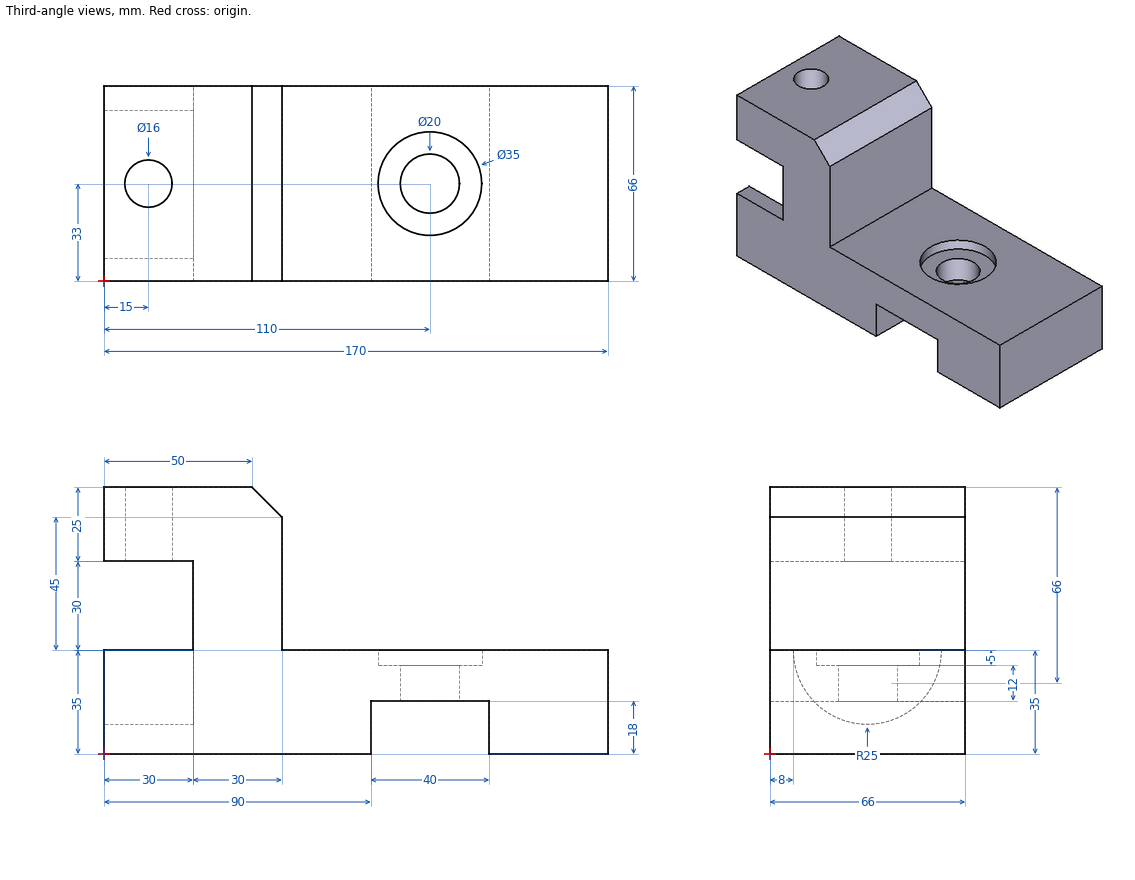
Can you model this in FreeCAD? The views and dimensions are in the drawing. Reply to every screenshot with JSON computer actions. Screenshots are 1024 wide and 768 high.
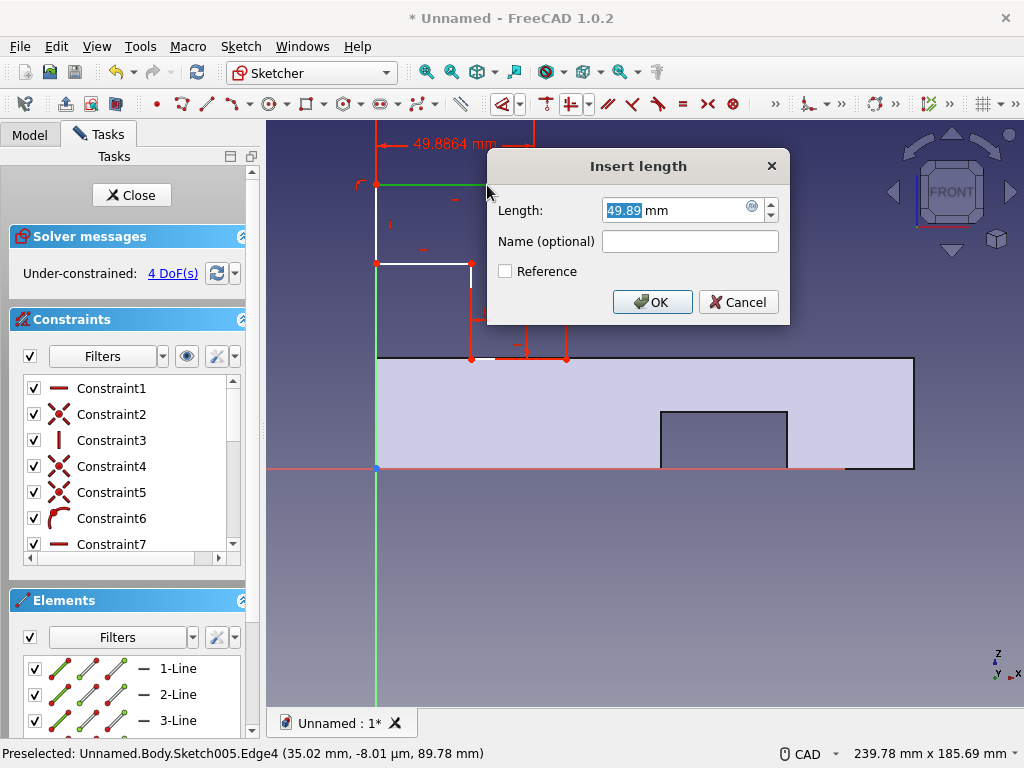
{"action": "type", "text": "50"}
{"action": "key", "text": "Return"}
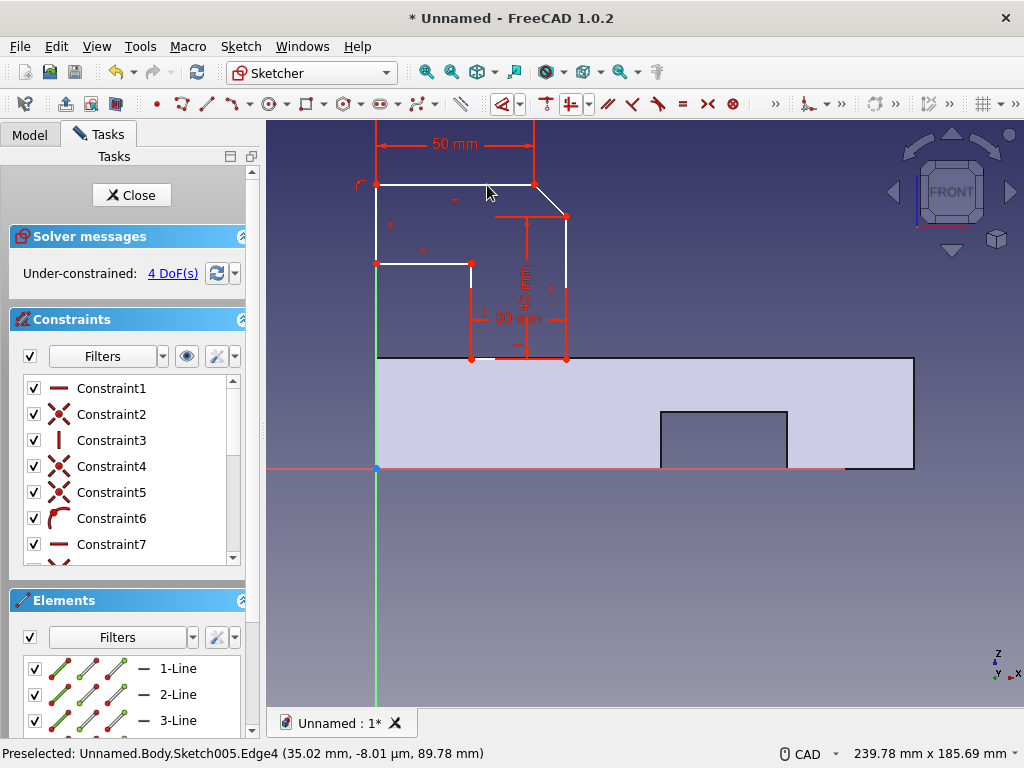
{"action": "left_click", "coordinate": [376, 209]}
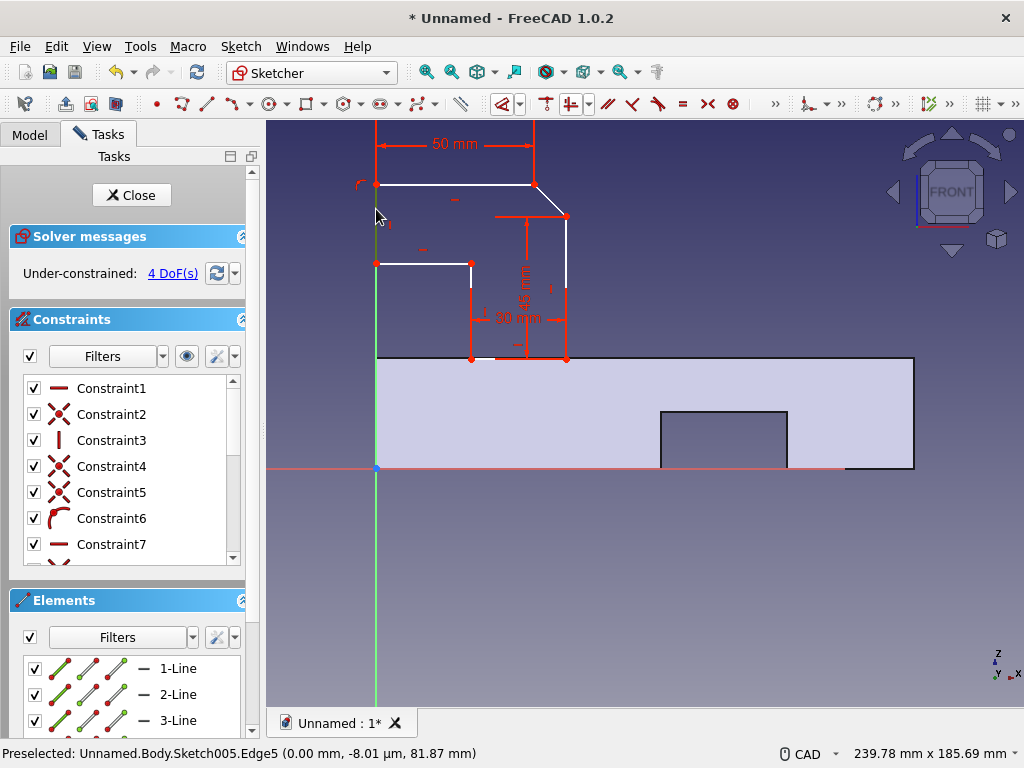
{"action": "key", "text": "i"}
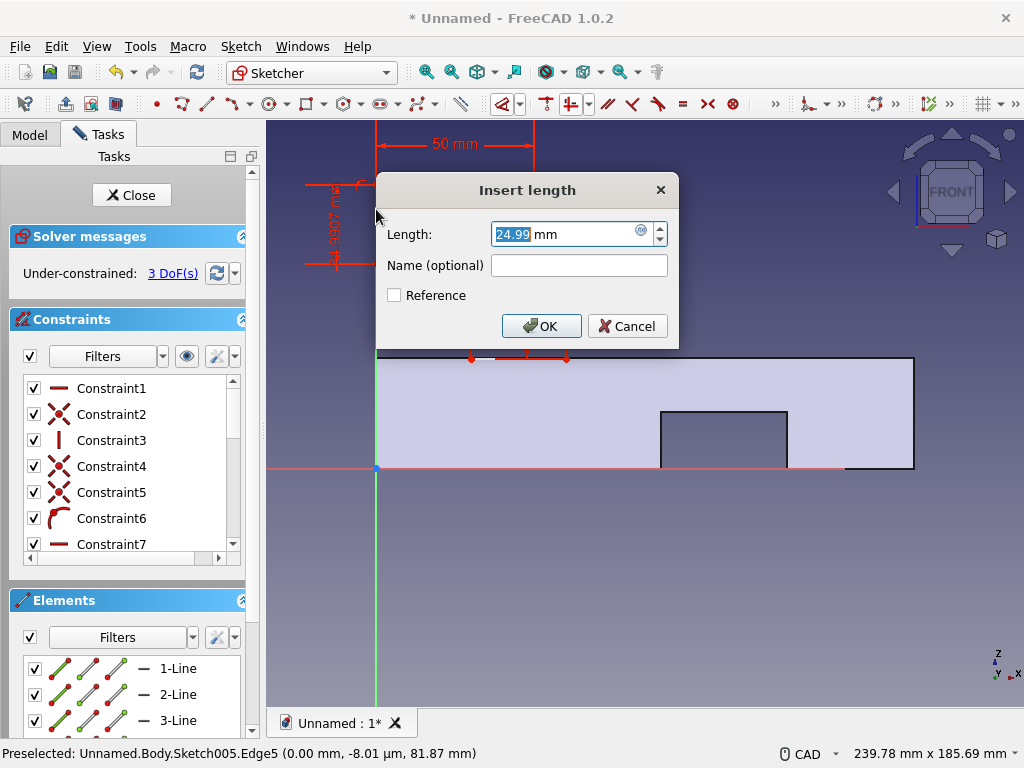
{"action": "type", "text": "25"}
{"action": "key", "text": "Return"}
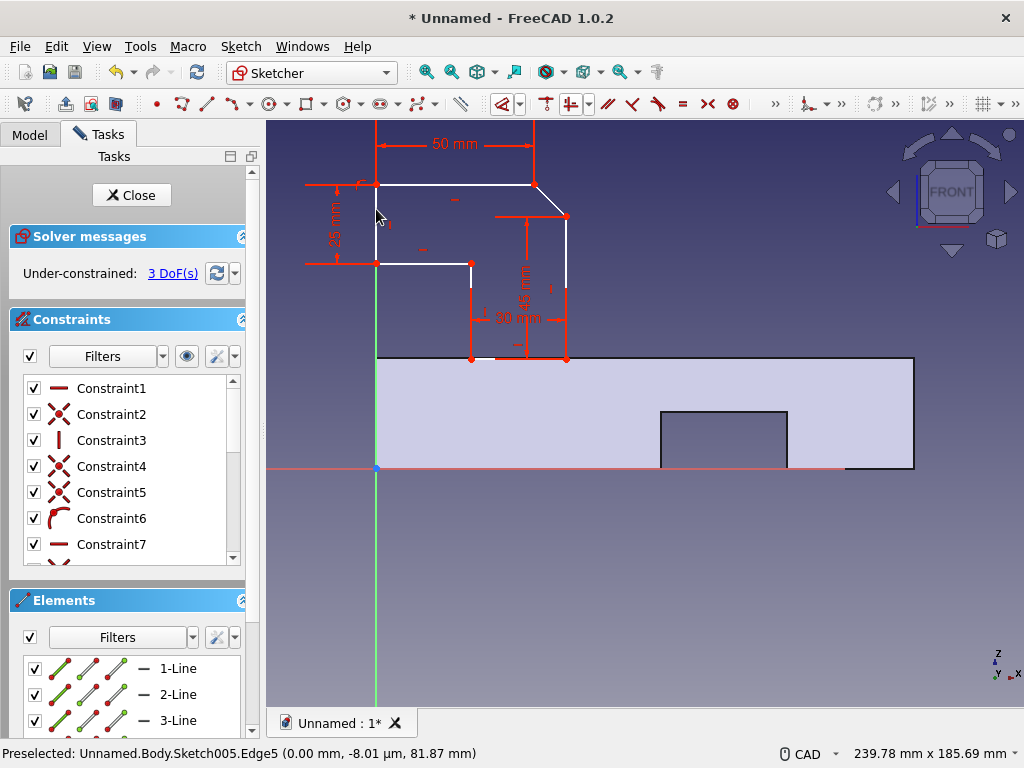
{"action": "left_click", "coordinate": [405, 264]}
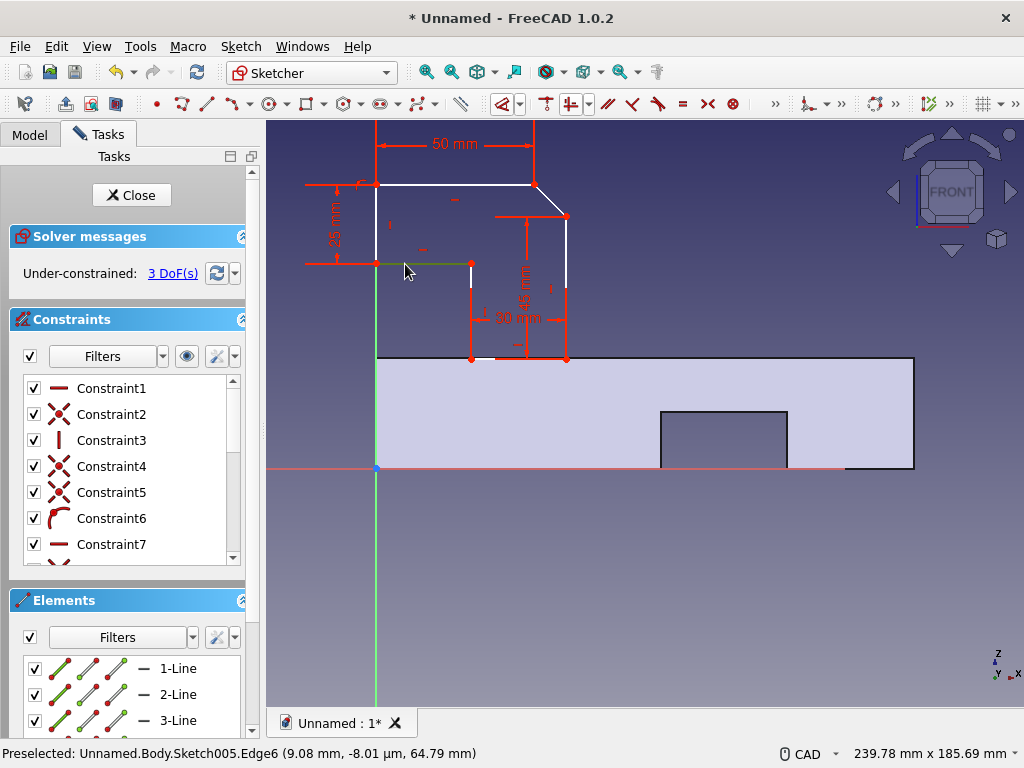
{"action": "left_click", "coordinate": [520, 104]}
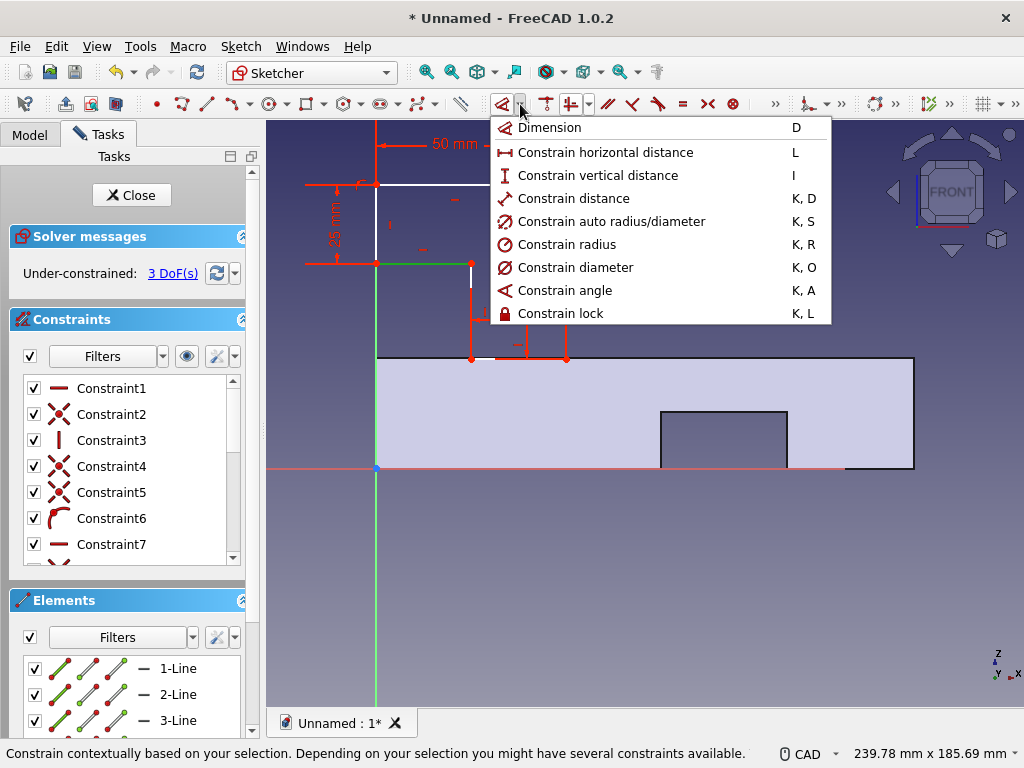
{"action": "left_click", "coordinate": [661, 152]}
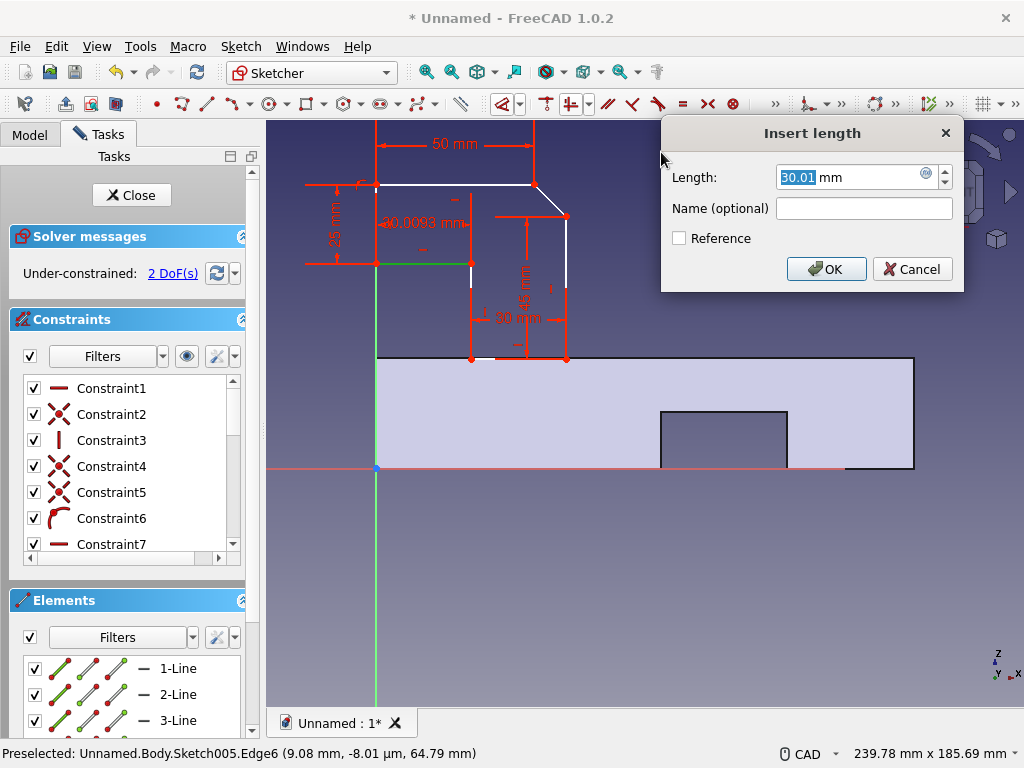
{"action": "type", "text": "30"}
{"action": "key", "text": "Return"}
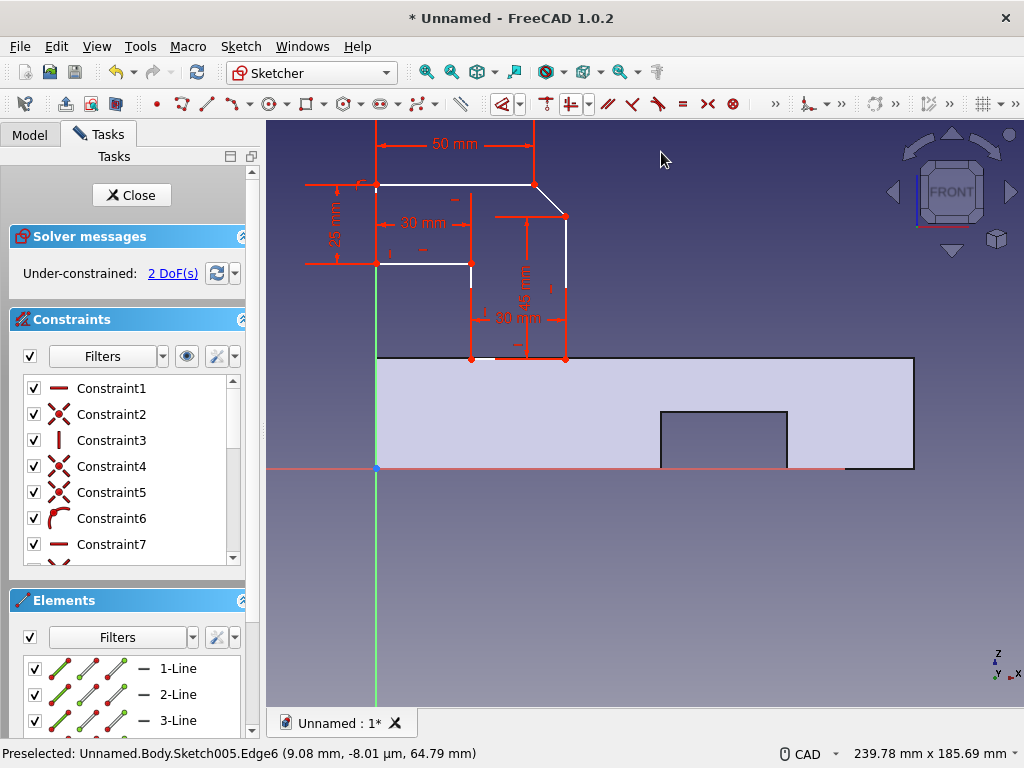
{"action": "left_click", "coordinate": [471, 293]}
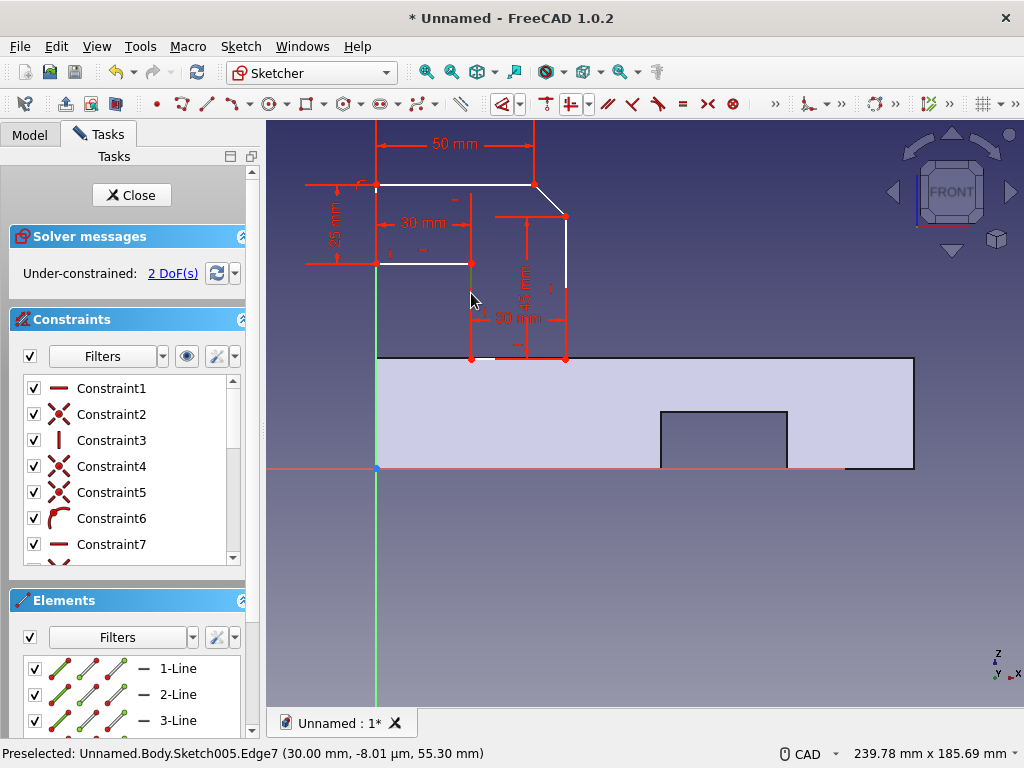
{"action": "key", "text": "i"}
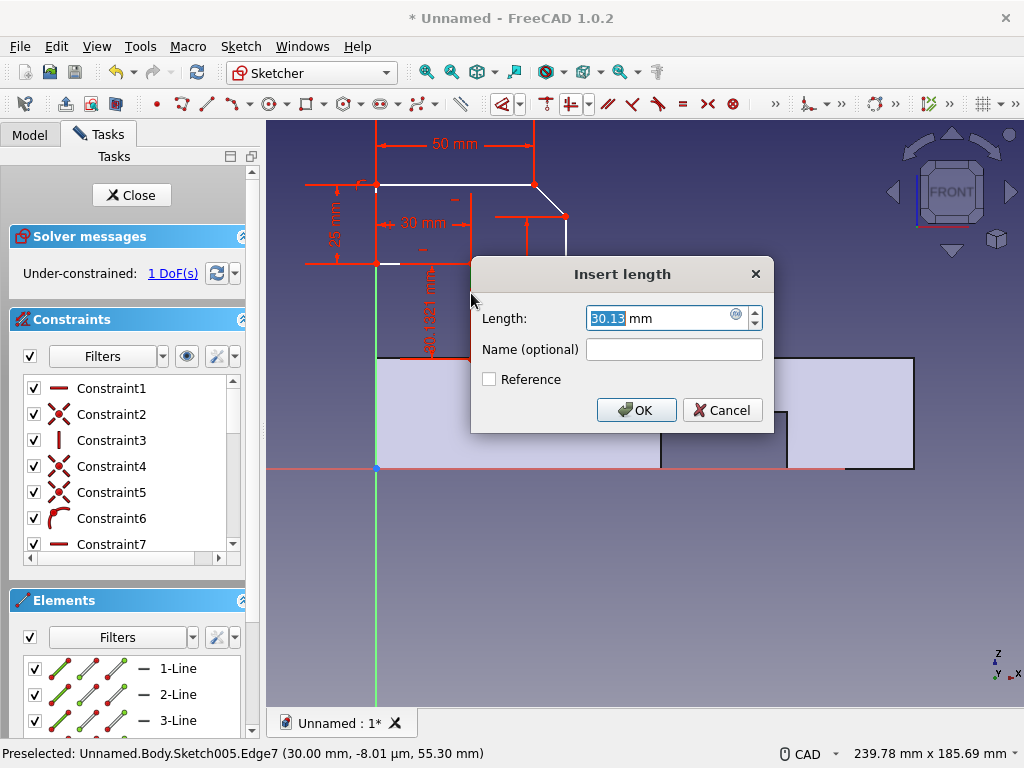
{"action": "type", "text": "30"}
{"action": "key", "text": "Return"}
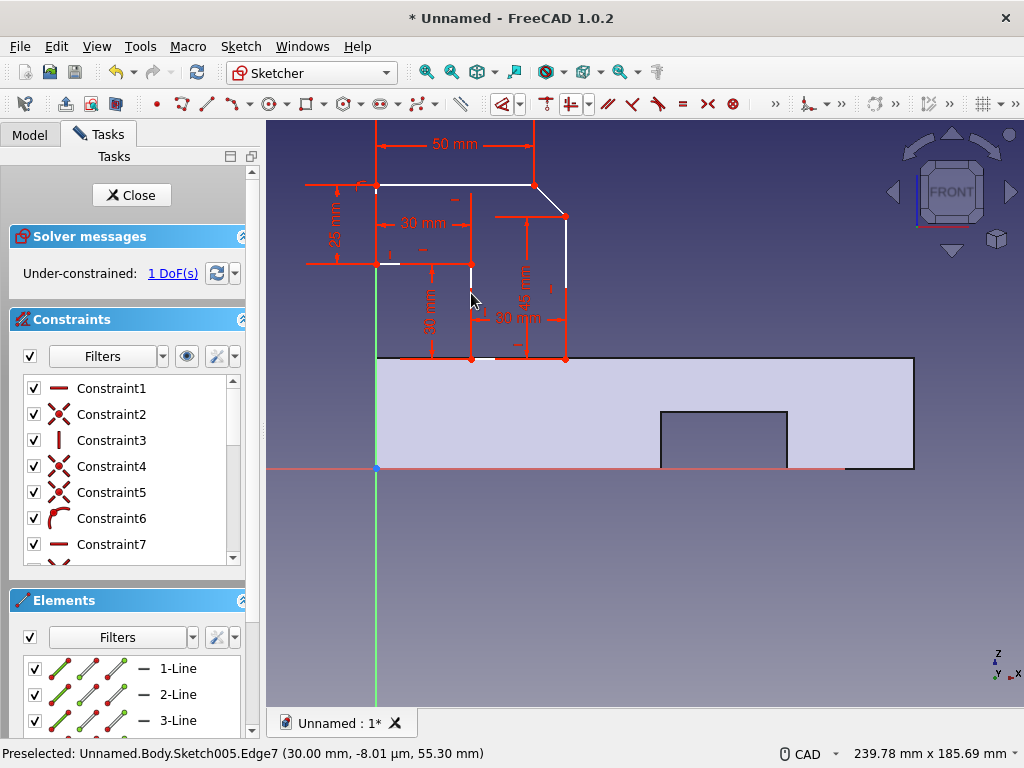
{"action": "left_click", "coordinate": [471, 359]}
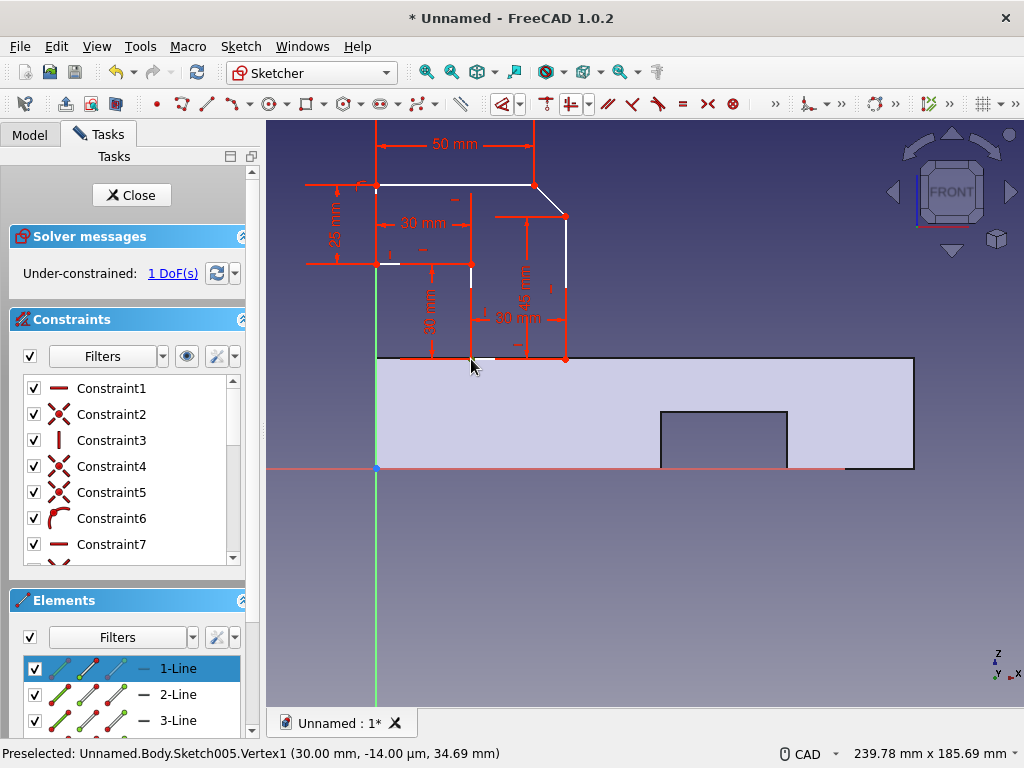
{"action": "left_click", "coordinate": [520, 104]}